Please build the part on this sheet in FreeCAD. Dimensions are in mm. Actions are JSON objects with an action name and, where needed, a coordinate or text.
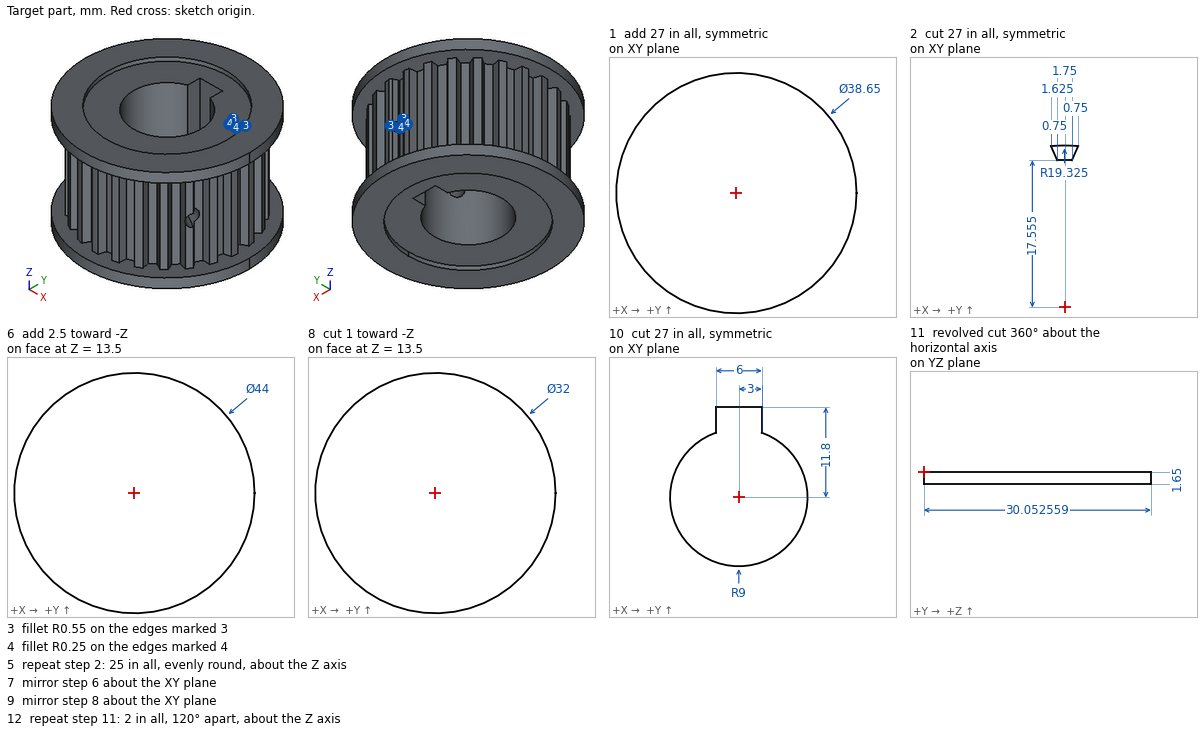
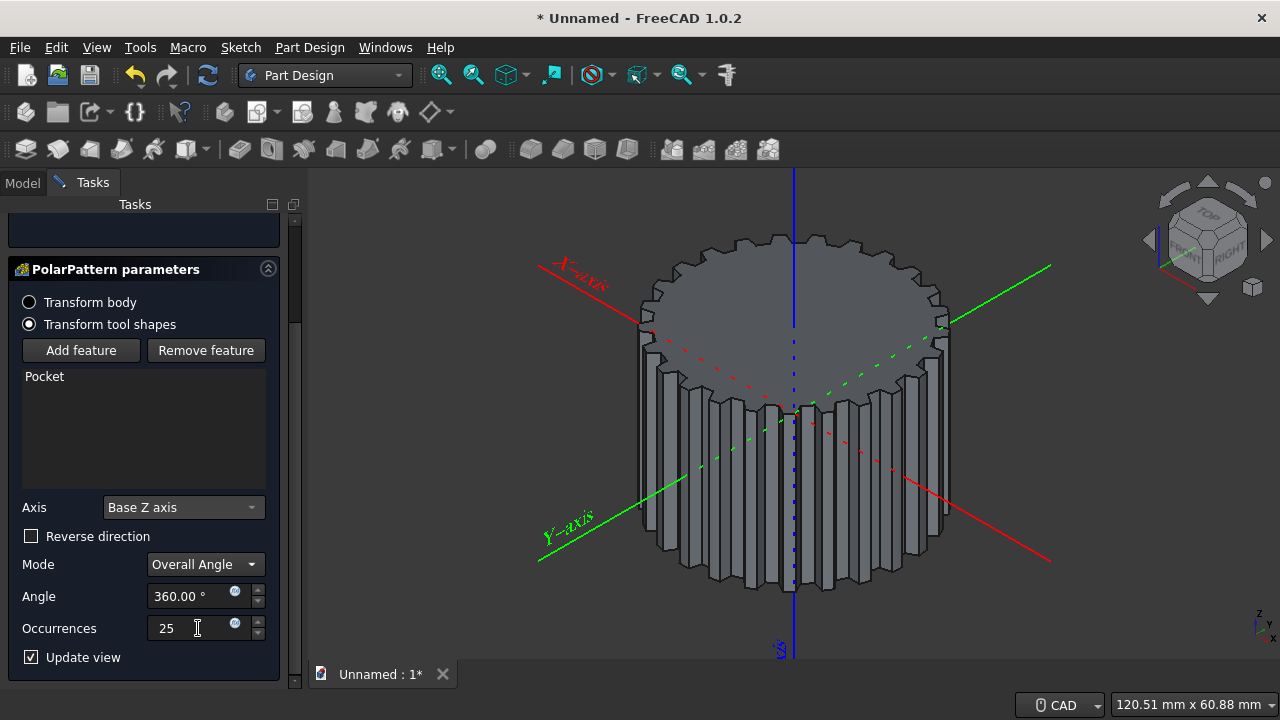
{"action": "scroll", "coordinate": [295, 451], "scroll_direction": "up", "scroll_amount": 3}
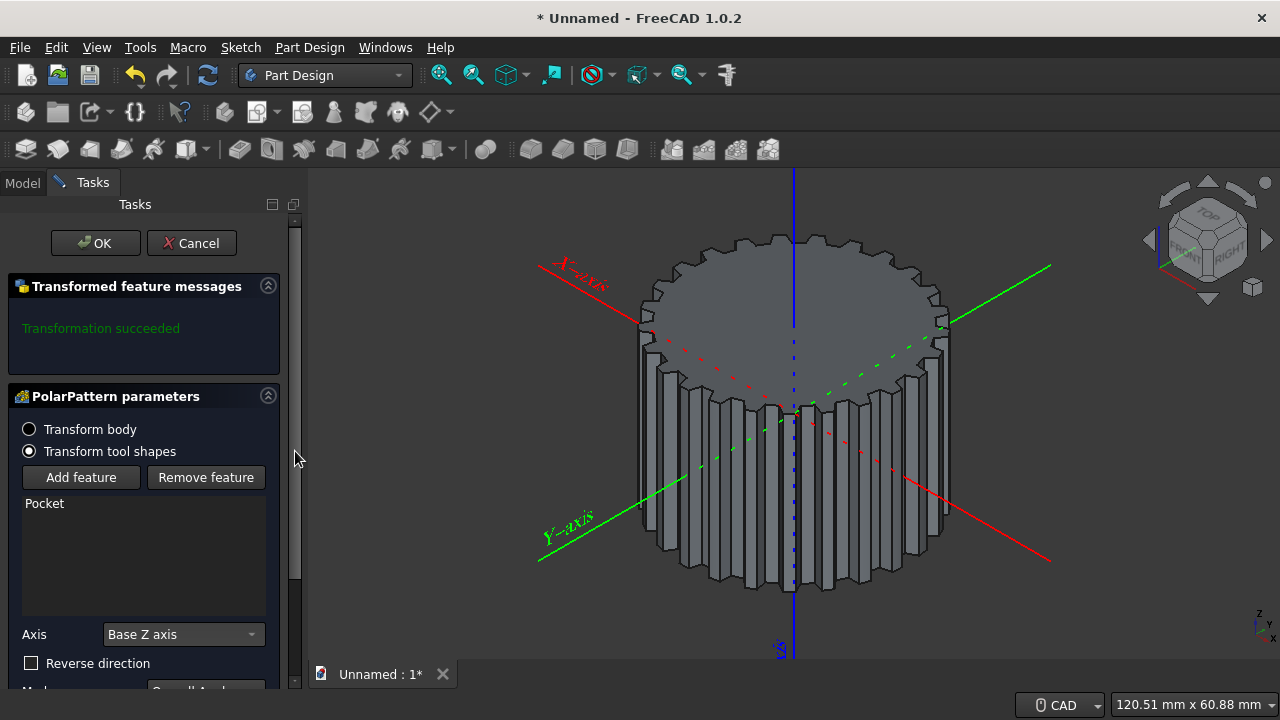
{"action": "left_click", "coordinate": [96, 243]}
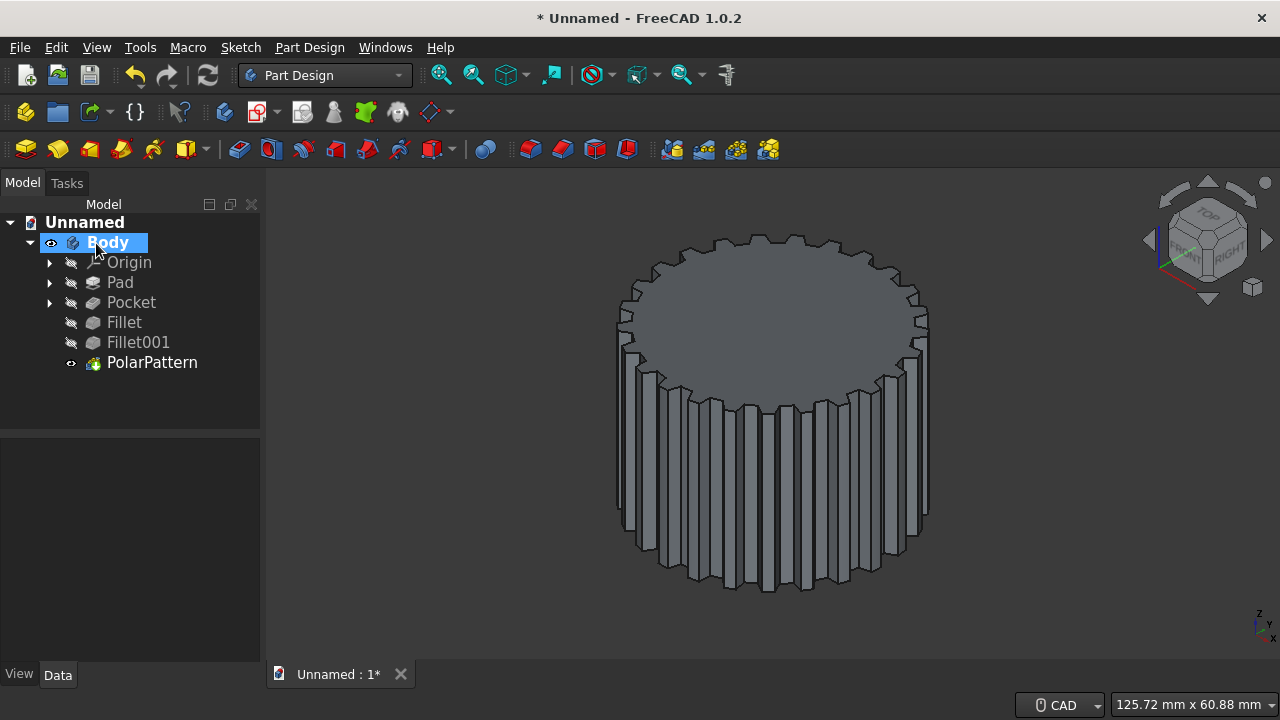
{"action": "left_click", "coordinate": [773, 324]}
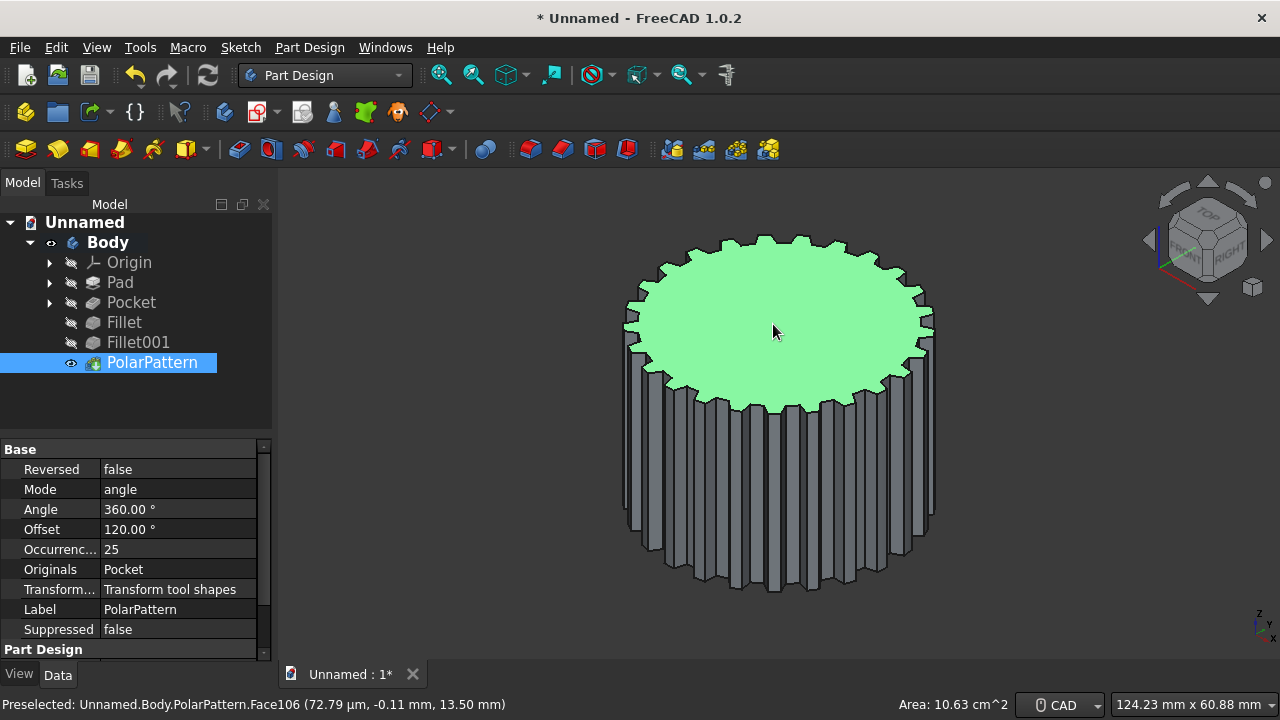
{"action": "left_click", "coordinate": [258, 112]}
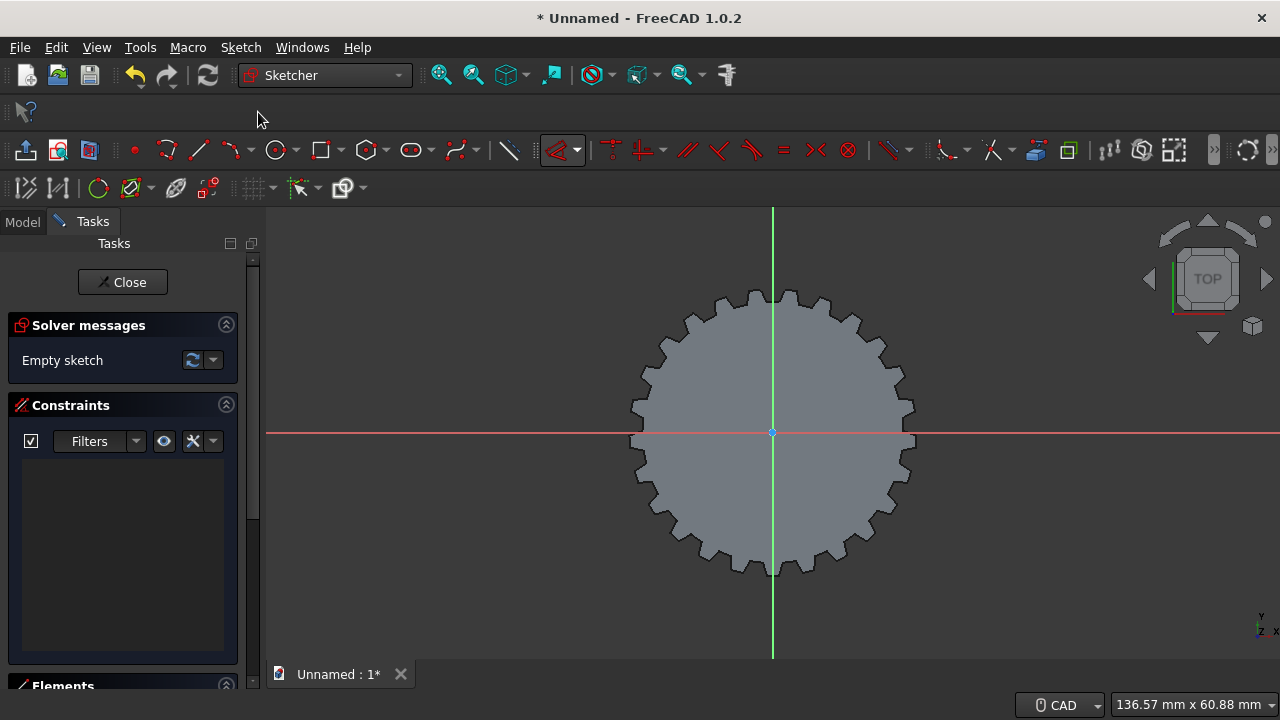
{"action": "left_click", "coordinate": [276, 150]}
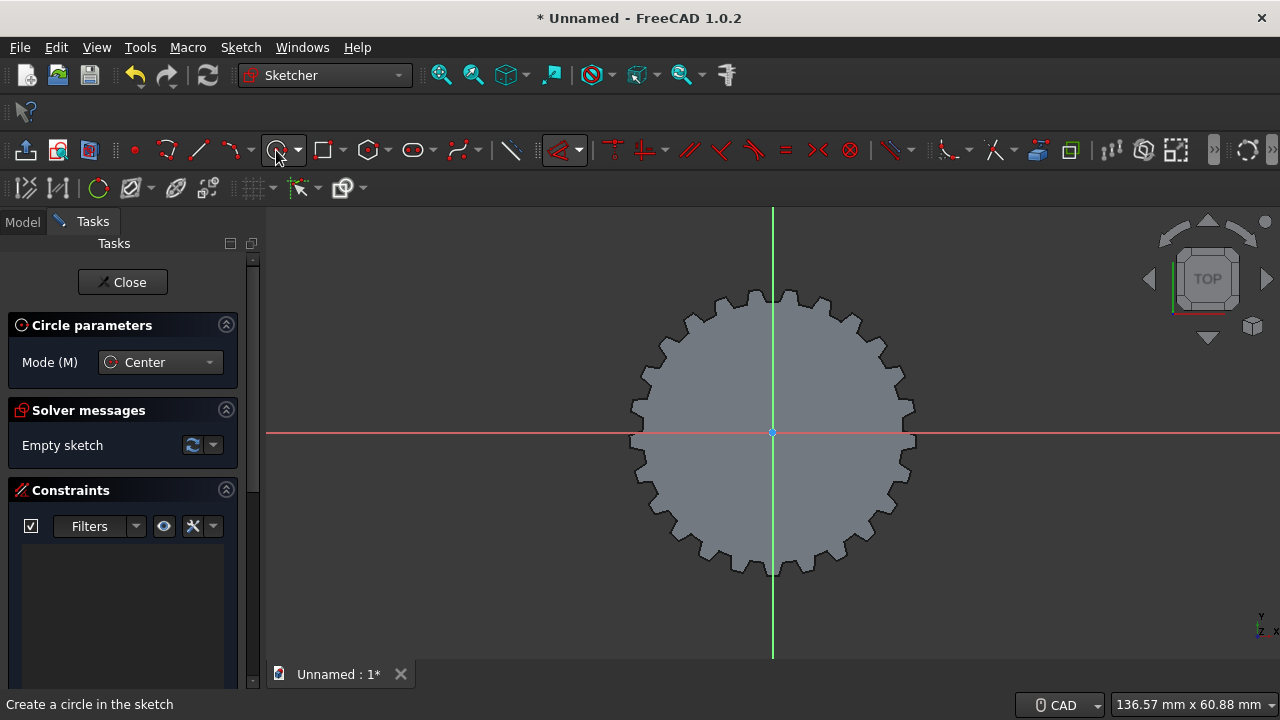
{"action": "left_click", "coordinate": [773, 433]}
{"action": "mouse_move", "coordinate": [888, 317]}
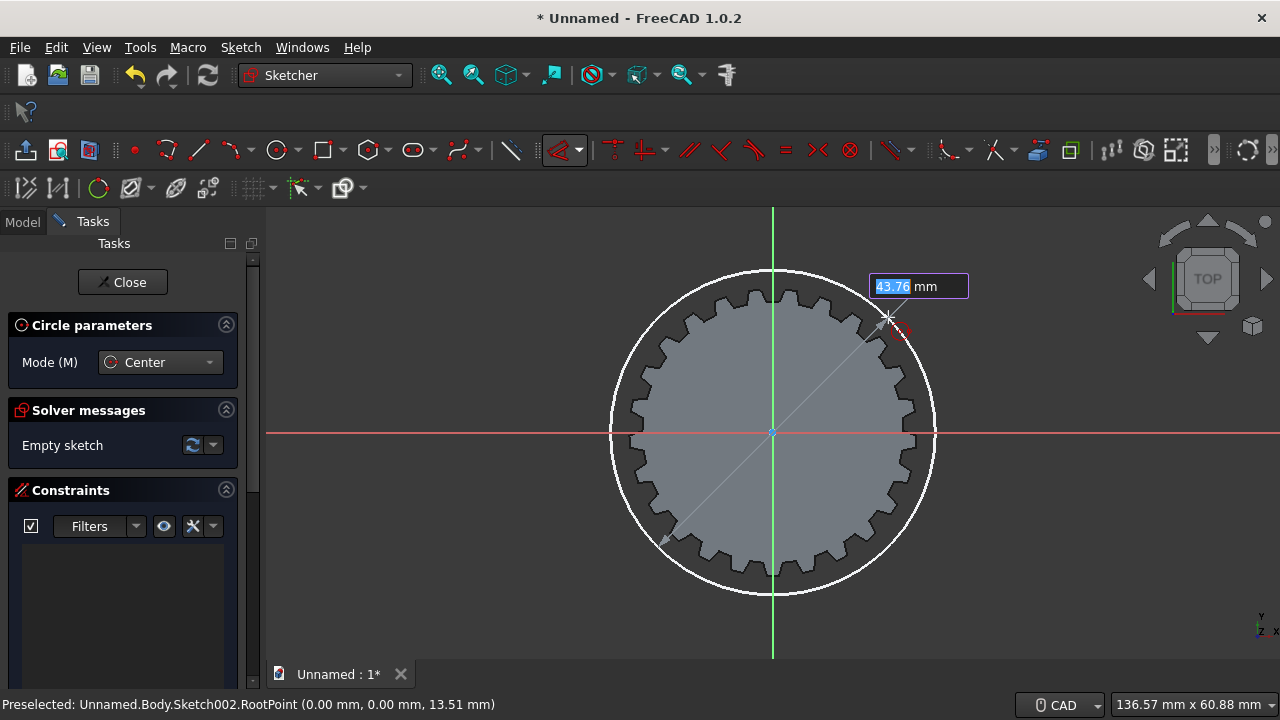
{"action": "type", "text": "44"}
{"action": "key", "text": "Return"}
{"action": "key", "text": "Escape"}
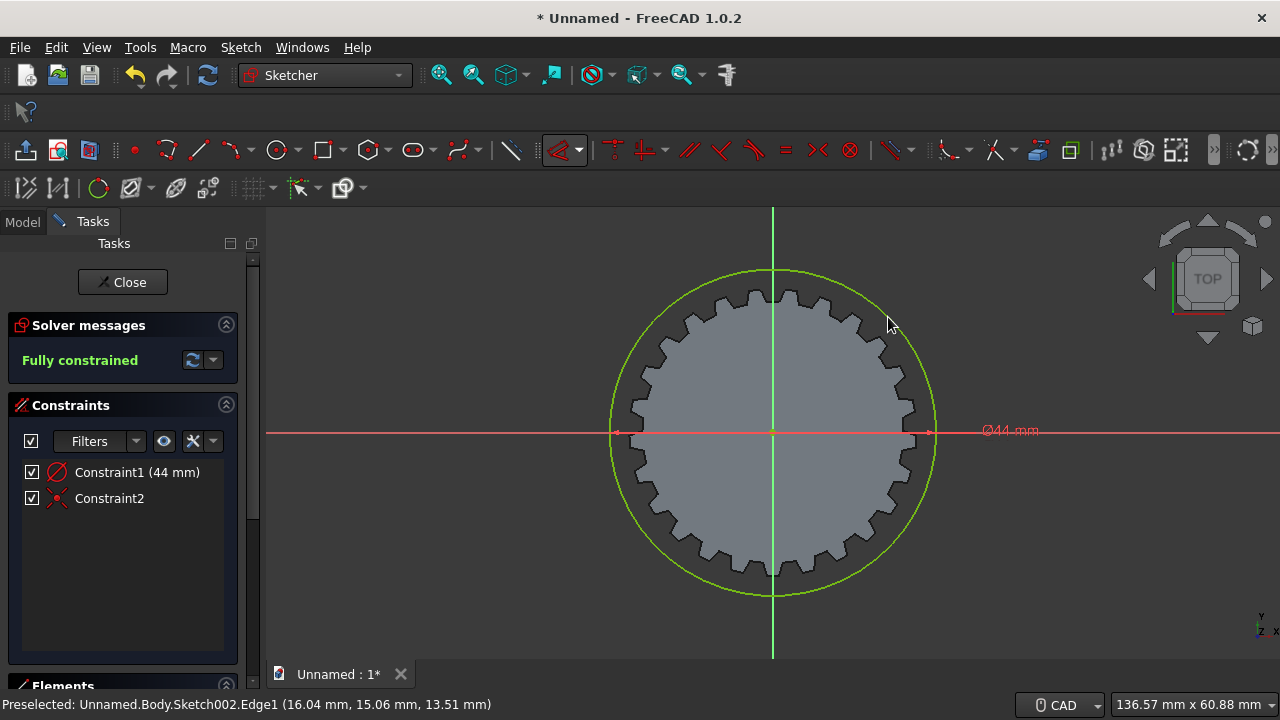
{"action": "left_click", "coordinate": [123, 282]}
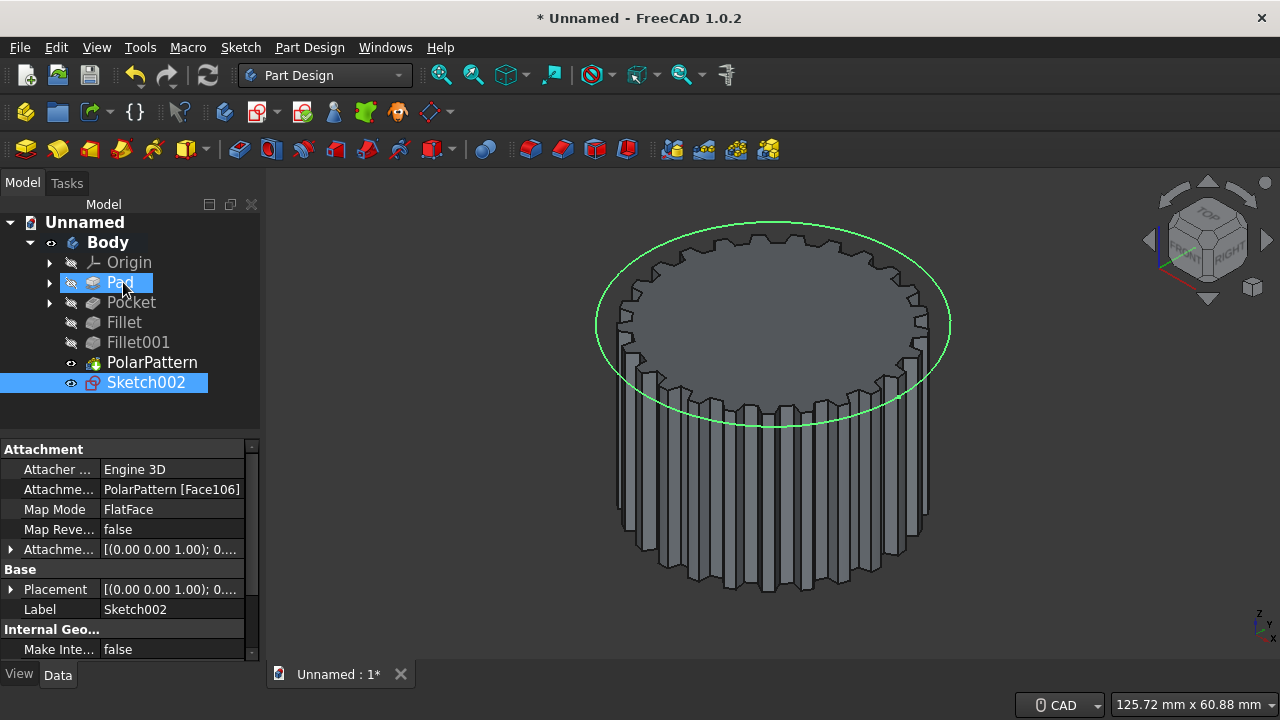
{"action": "left_click", "coordinate": [26, 150]}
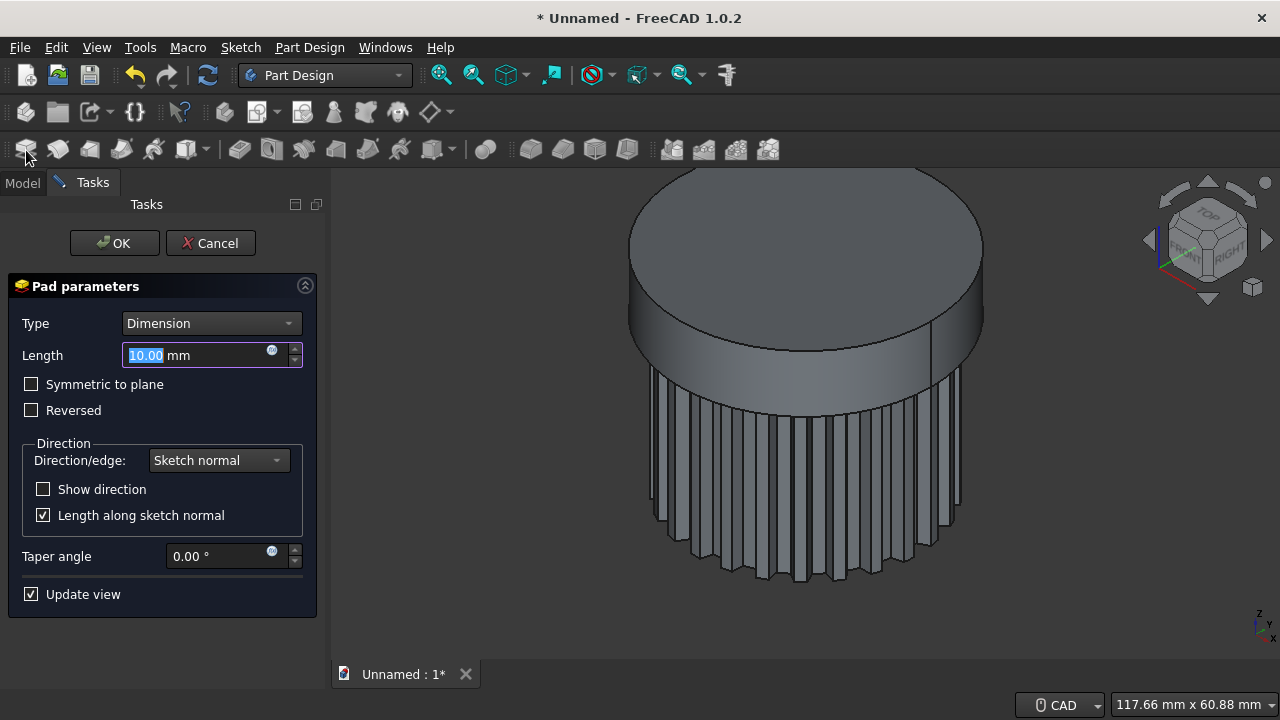
{"action": "type", "text": "2.5"}
{"action": "key", "text": "Tab"}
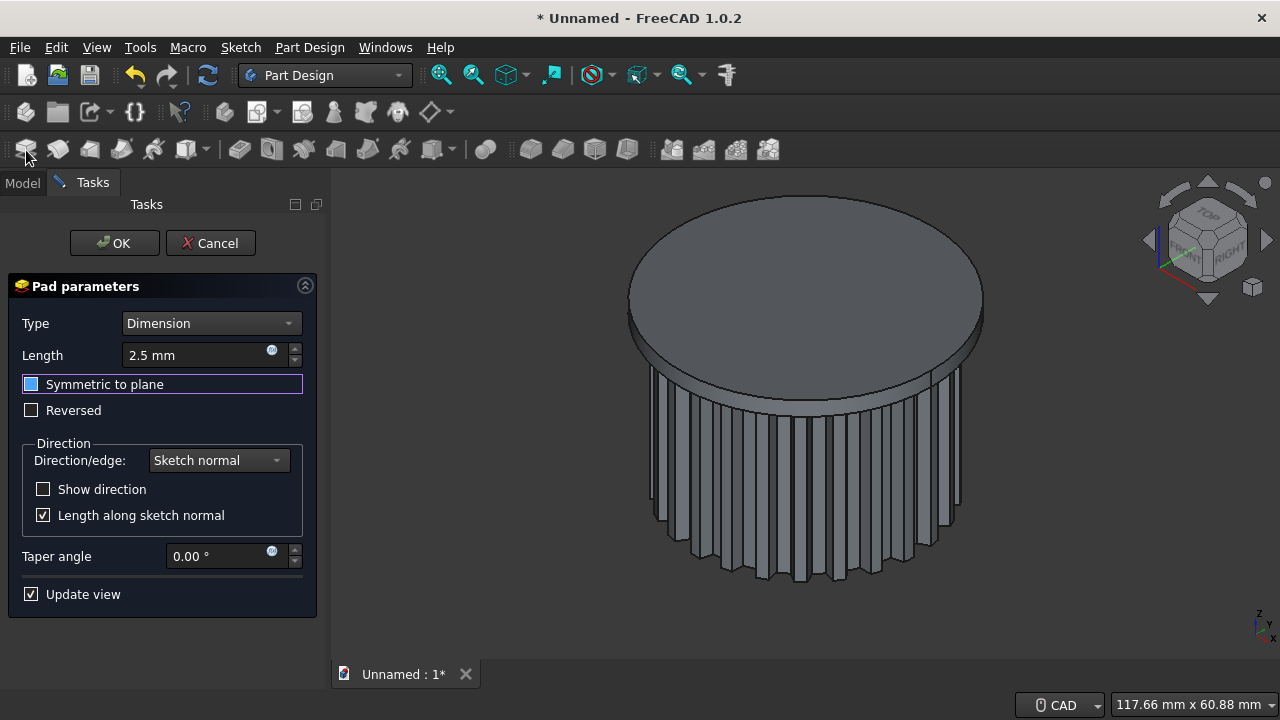
{"action": "left_click", "coordinate": [30, 410]}